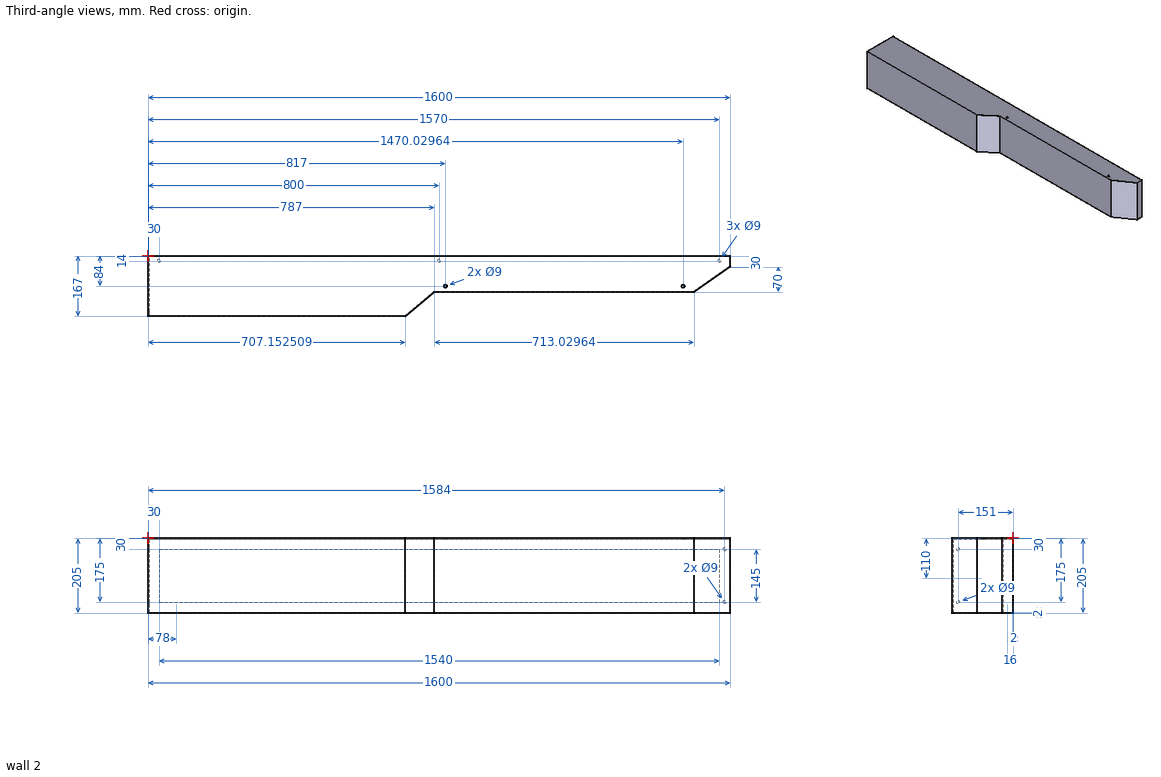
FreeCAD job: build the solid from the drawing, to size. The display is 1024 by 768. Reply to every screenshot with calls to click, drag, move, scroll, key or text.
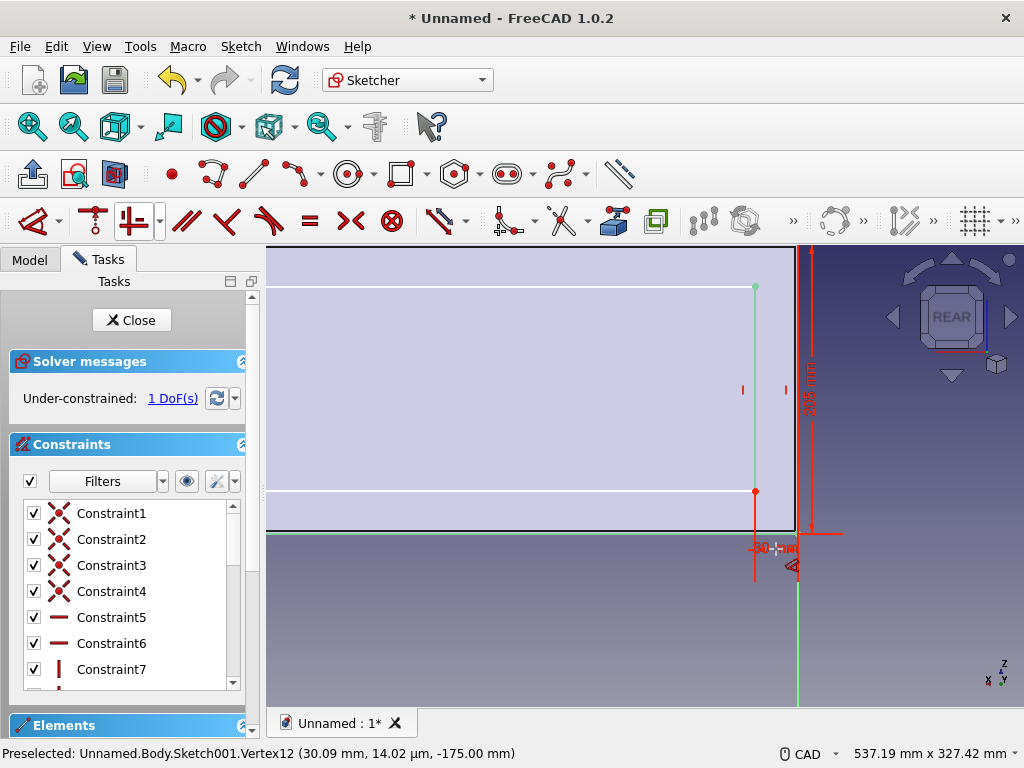
scroll(756, 493, down, 9)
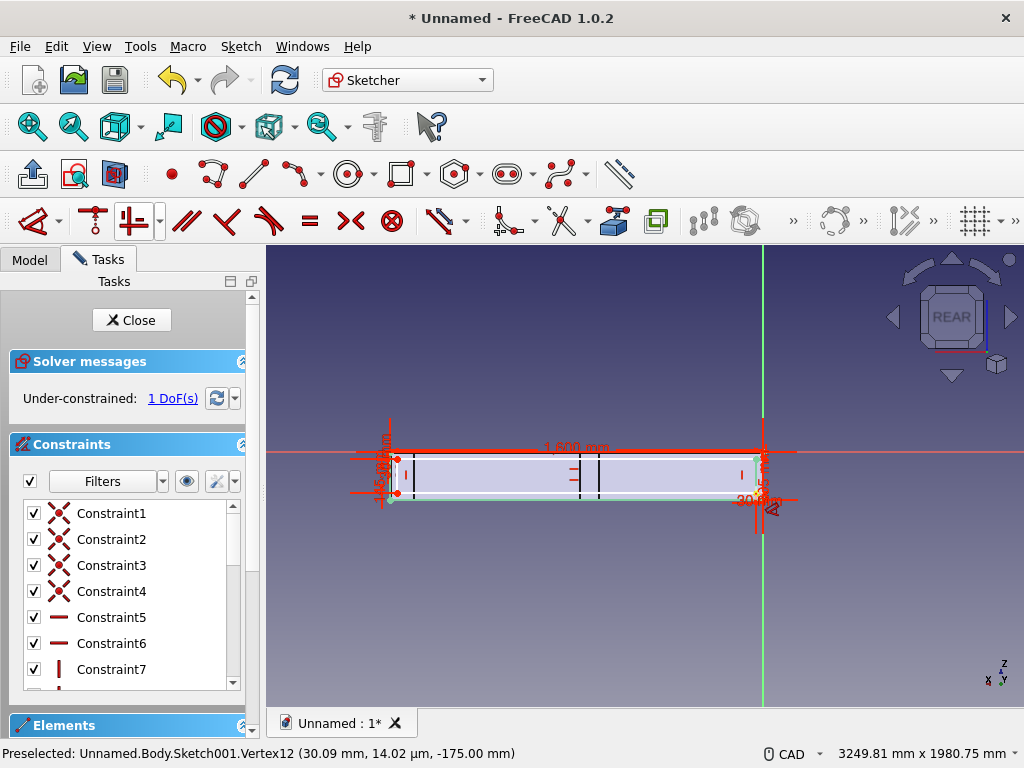
scroll(685, 493, up, 4)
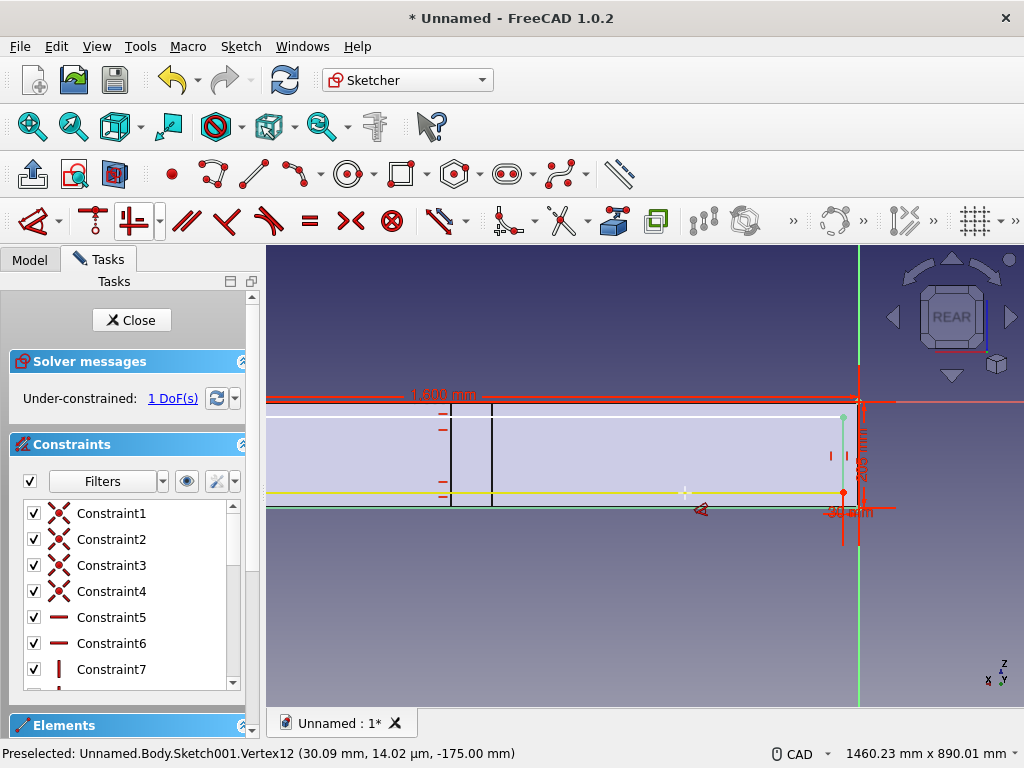
click(683, 493)
click(569, 527)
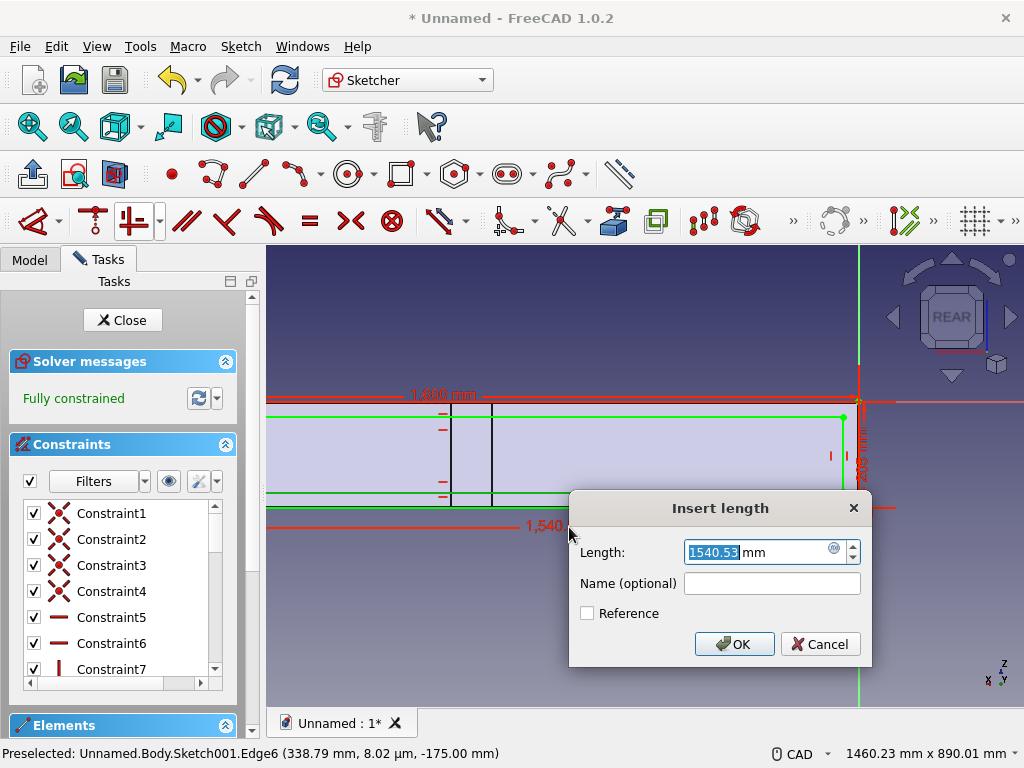
text(1540)
key(Return)
key(Escape)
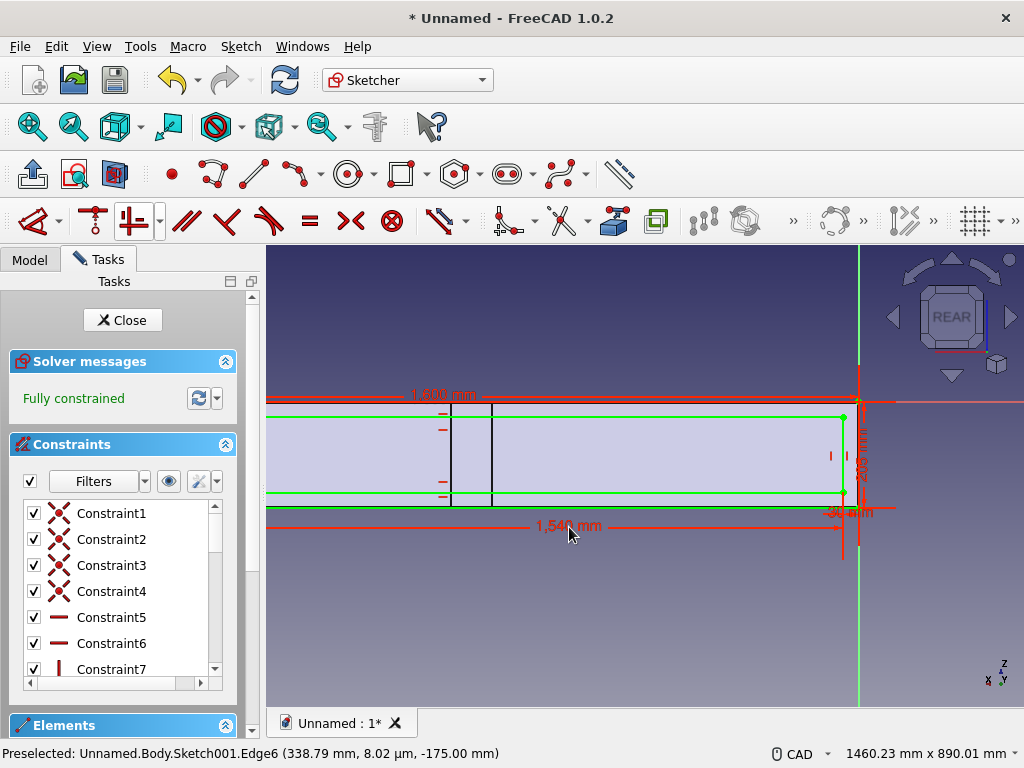
click(123, 320)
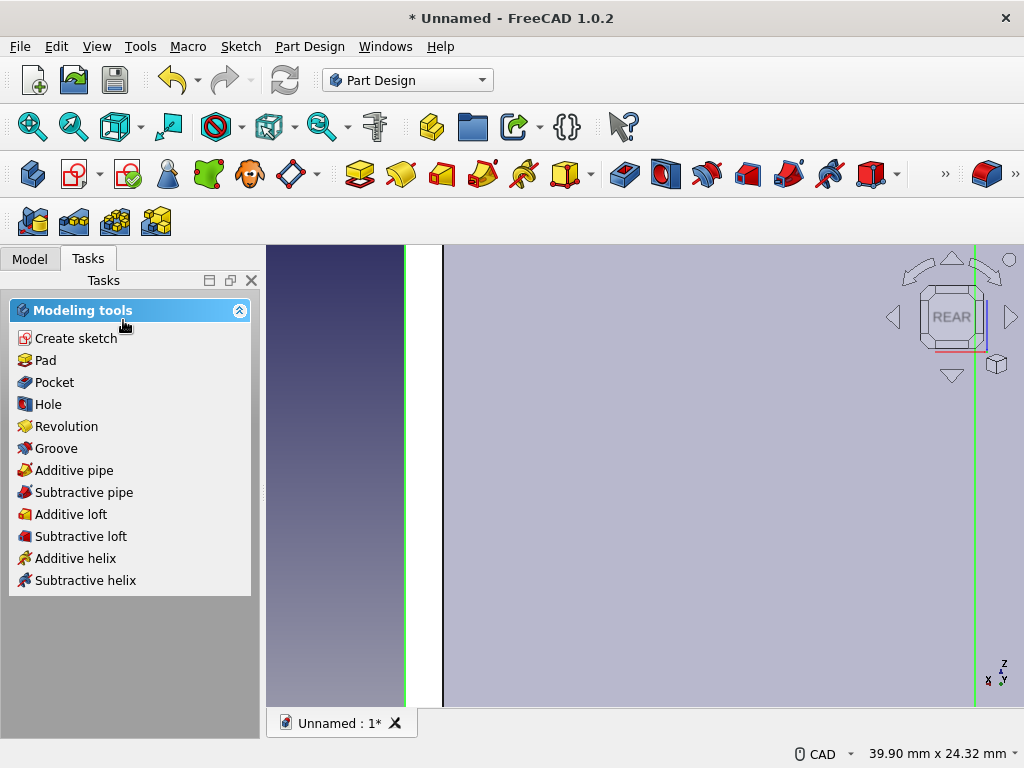
click(360, 174)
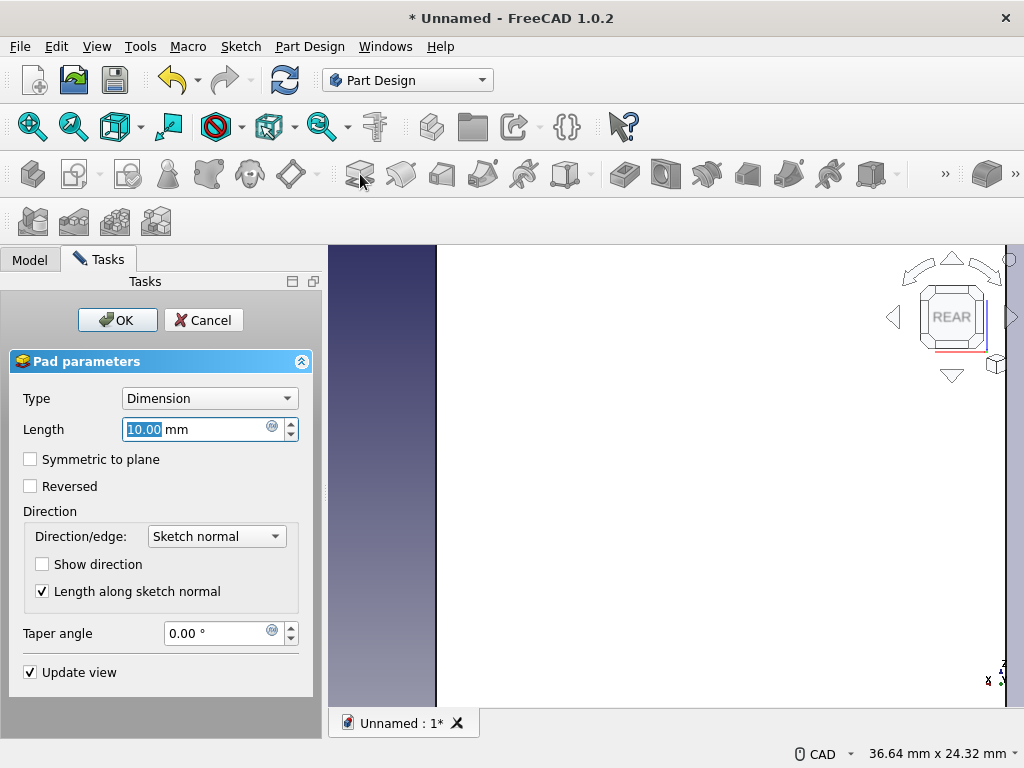
text(2)
key(Tab)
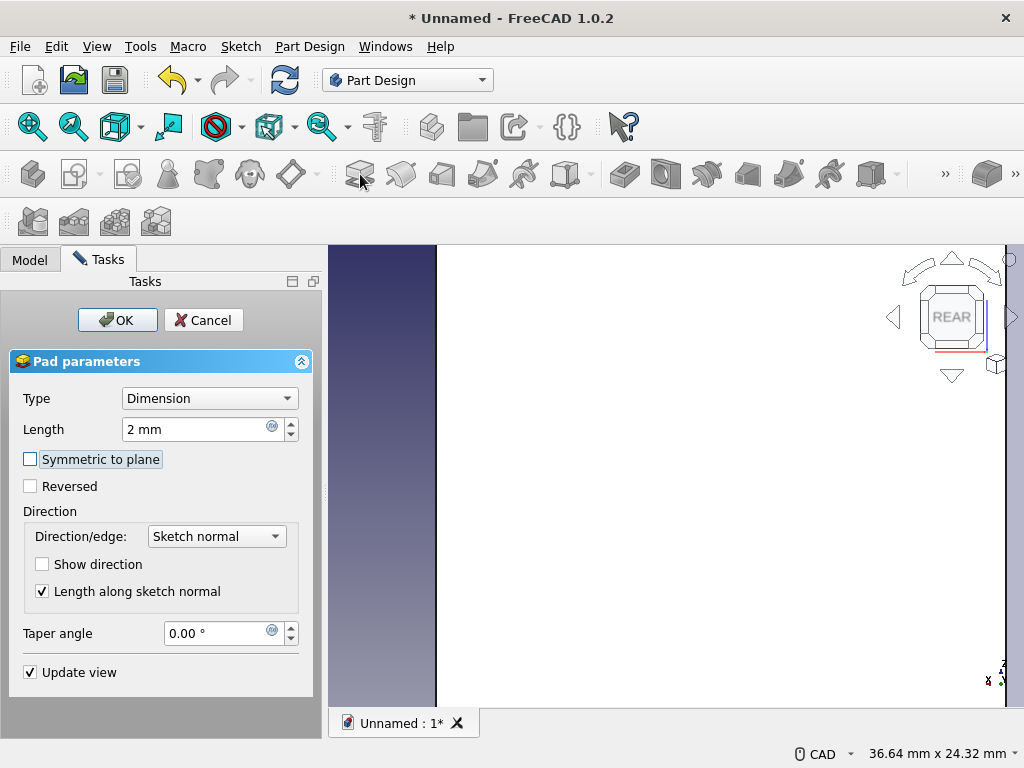
click(31, 486)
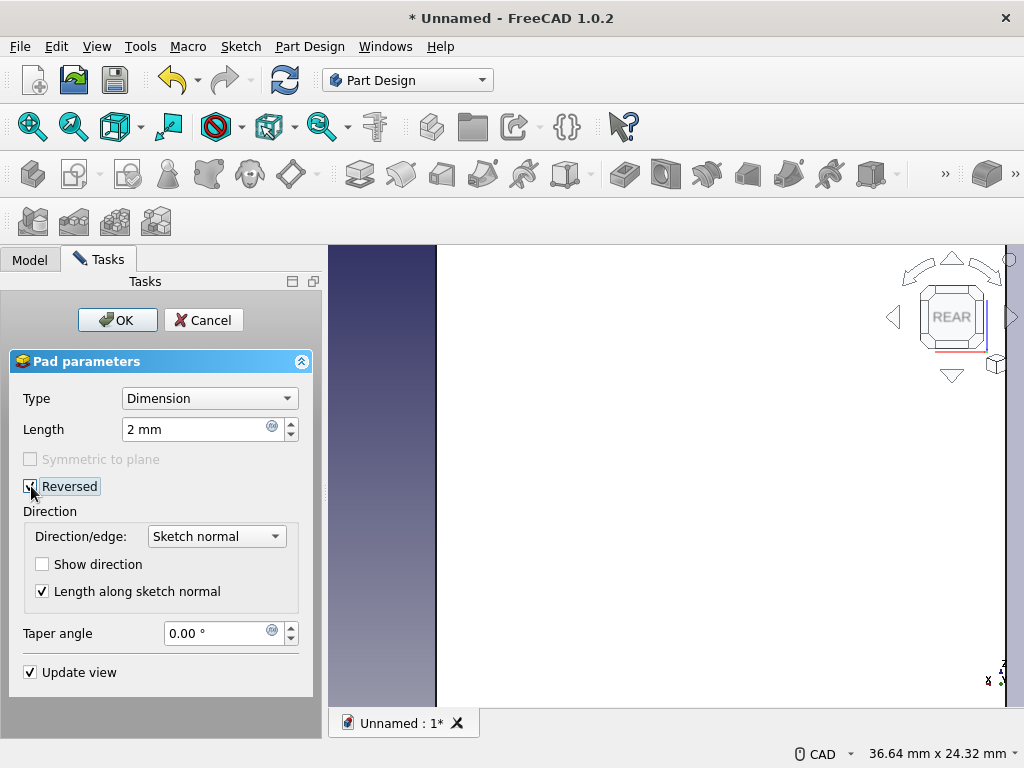
click(118, 320)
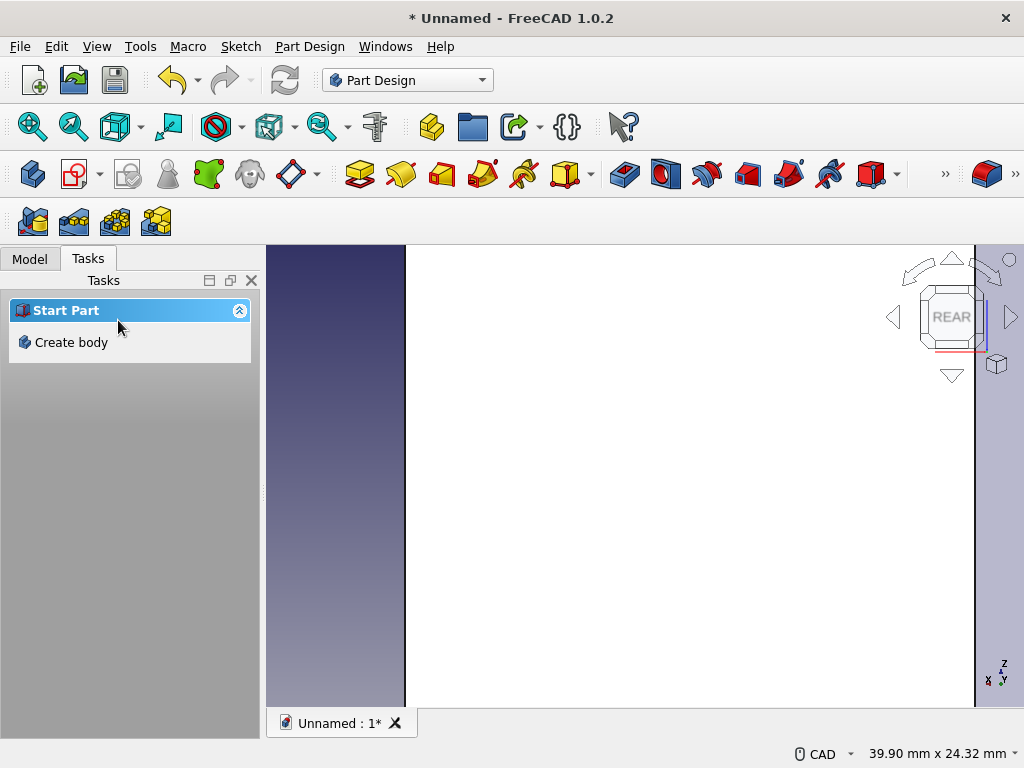
key(v)
key(f)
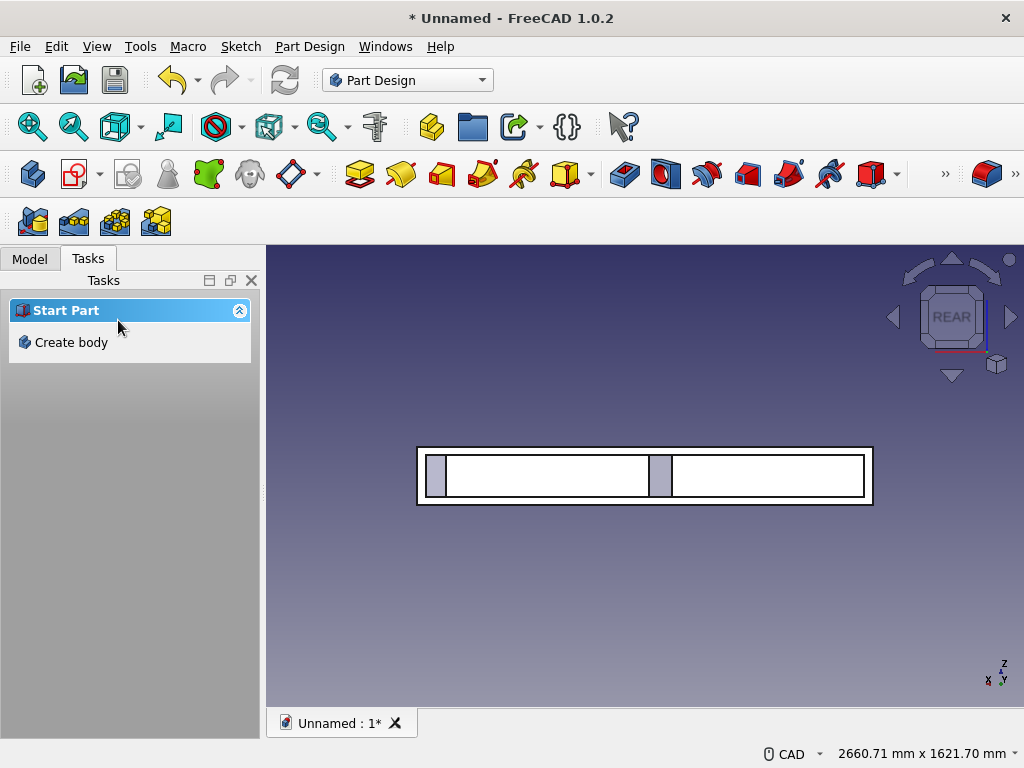
key(5)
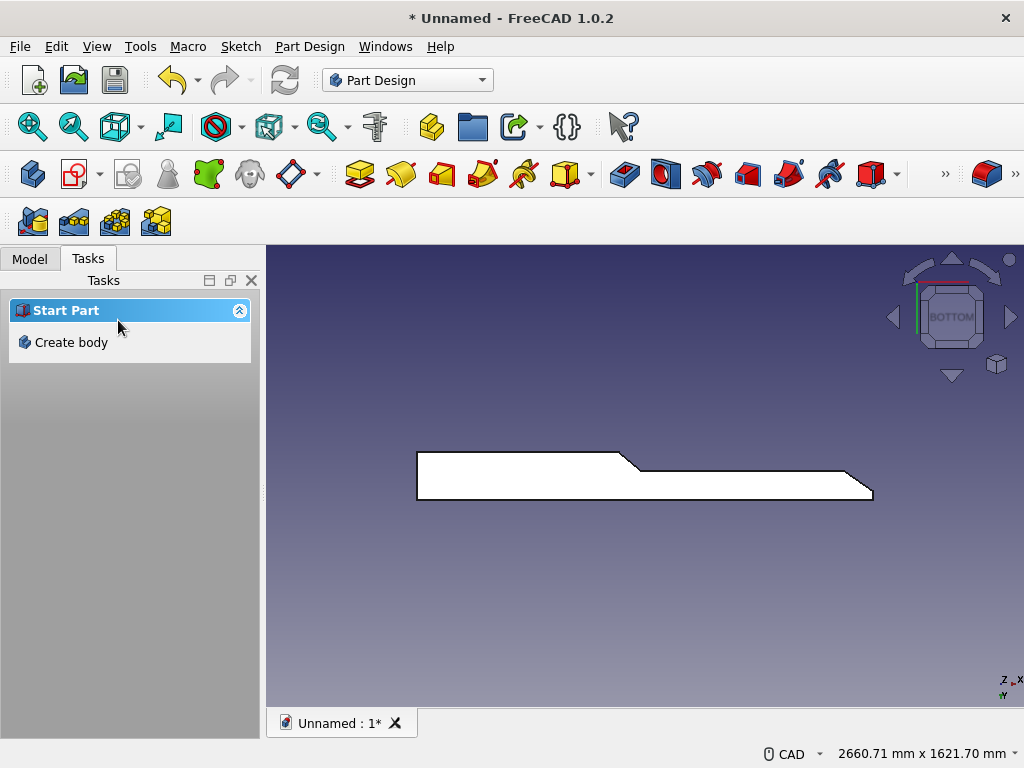
click(580, 475)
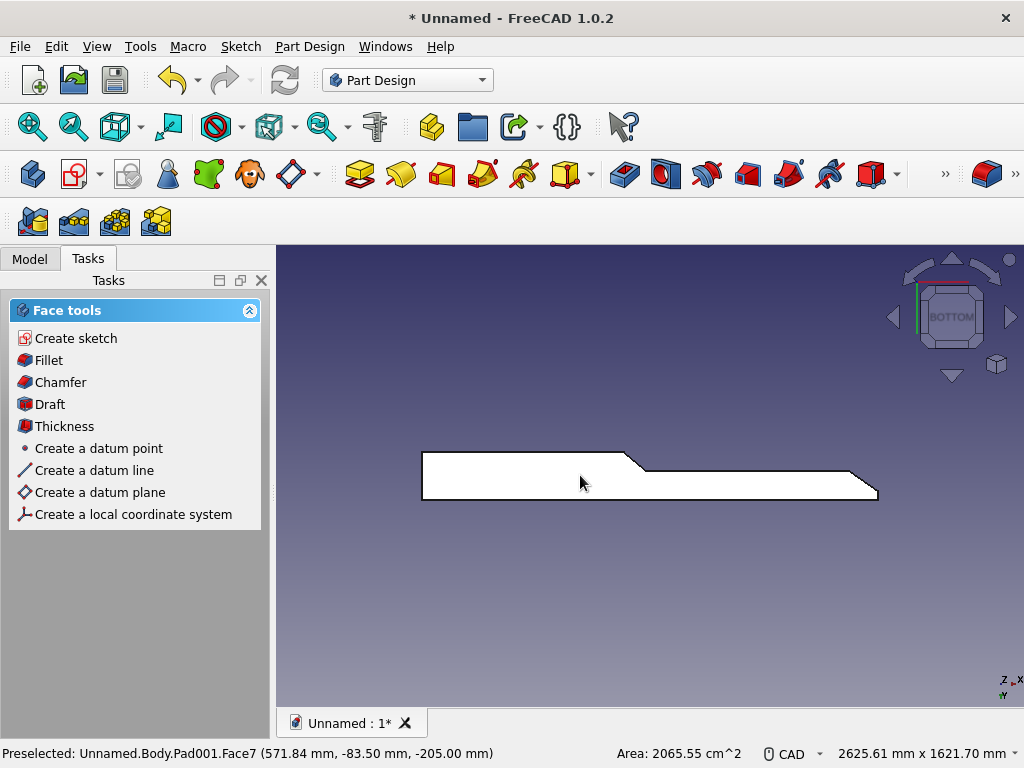
click(74, 174)